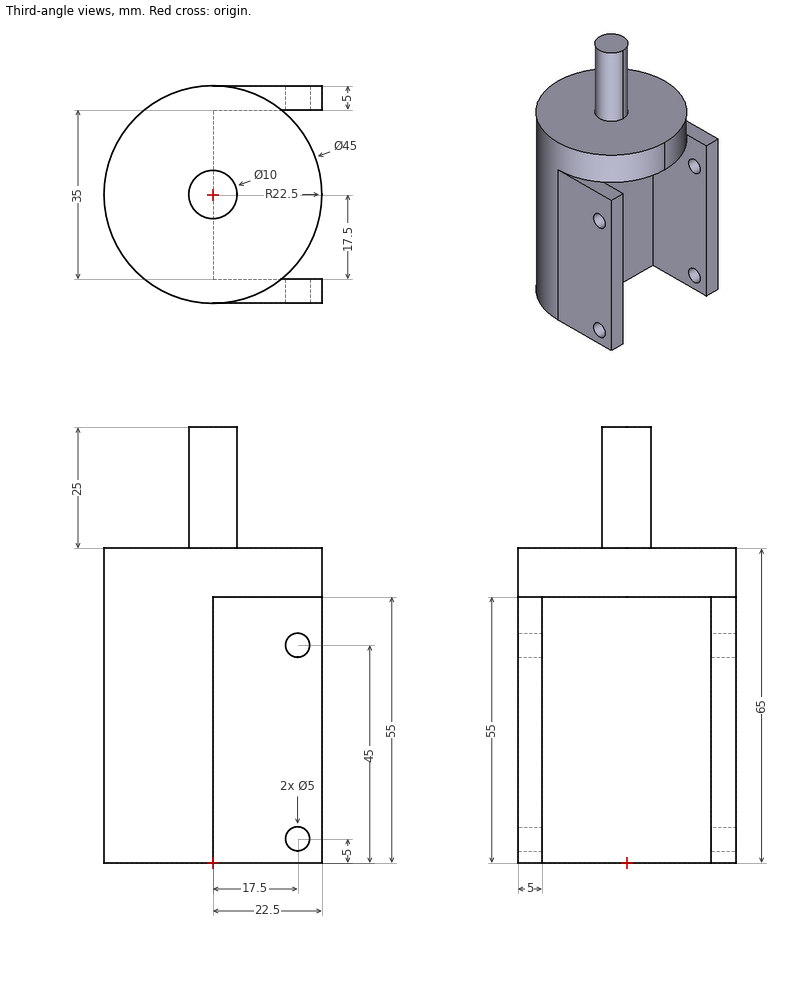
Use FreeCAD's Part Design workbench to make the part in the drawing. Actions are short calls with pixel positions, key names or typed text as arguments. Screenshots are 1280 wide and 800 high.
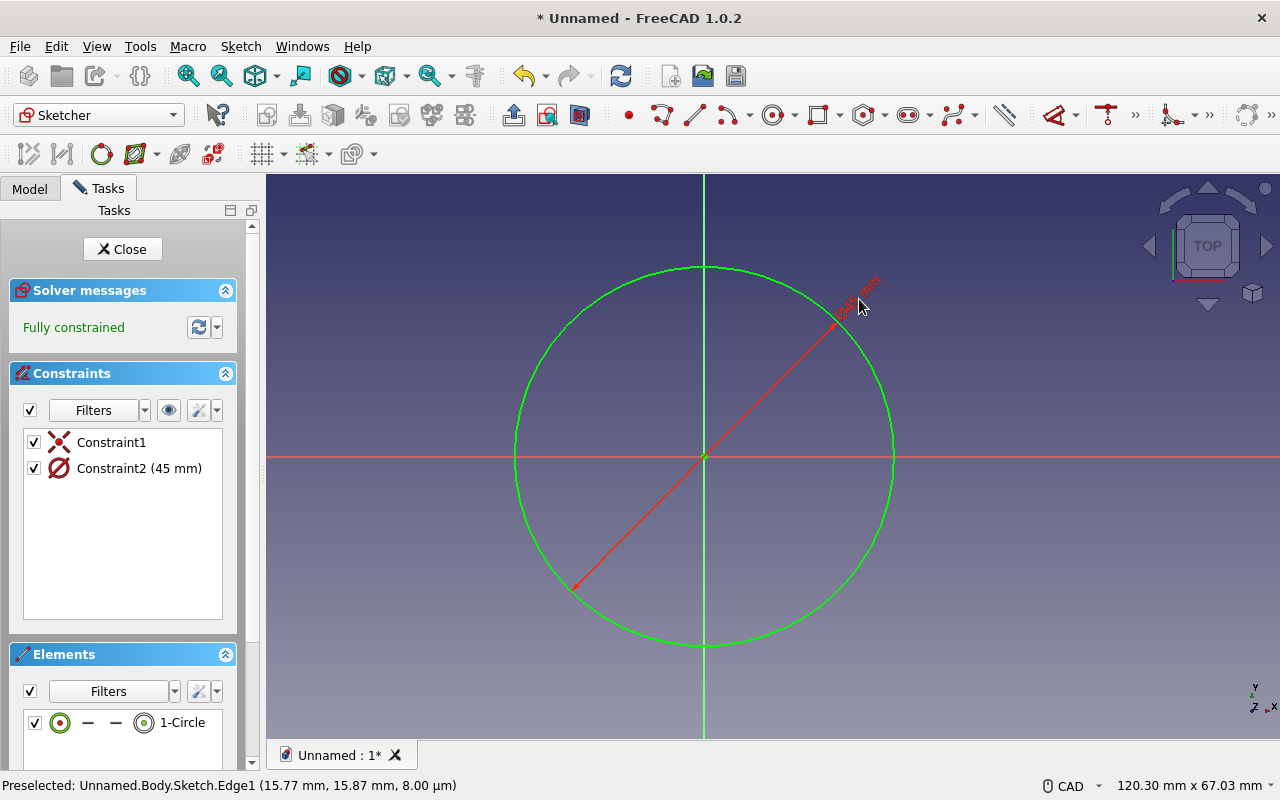
click(123, 249)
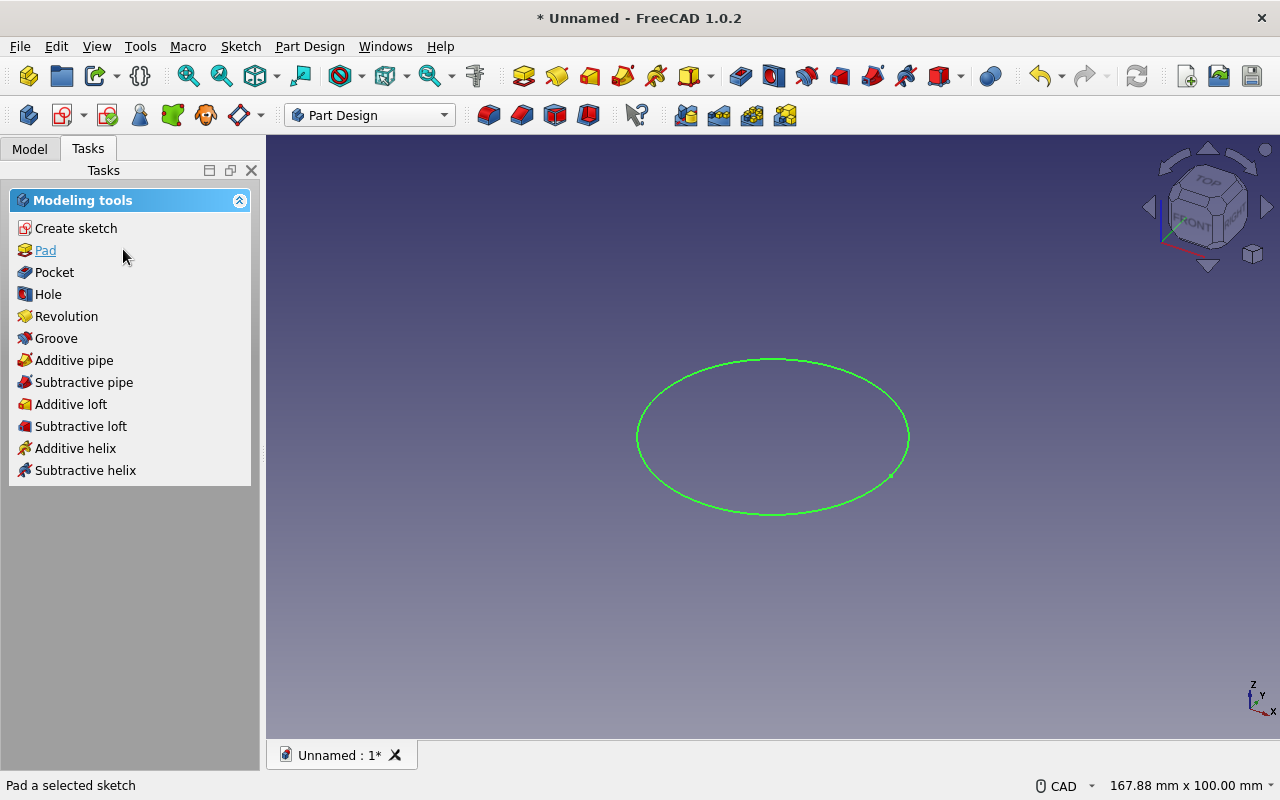
click(524, 76)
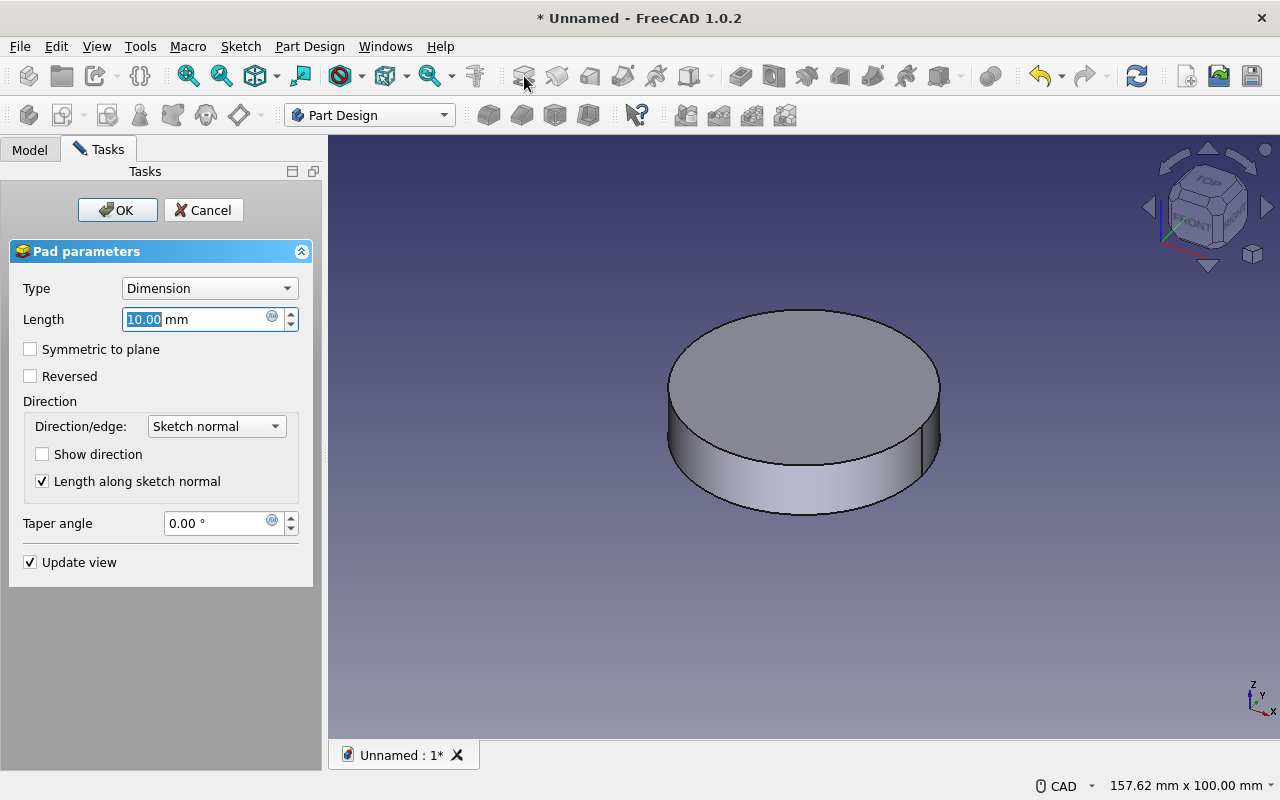
text(65)
key(Tab)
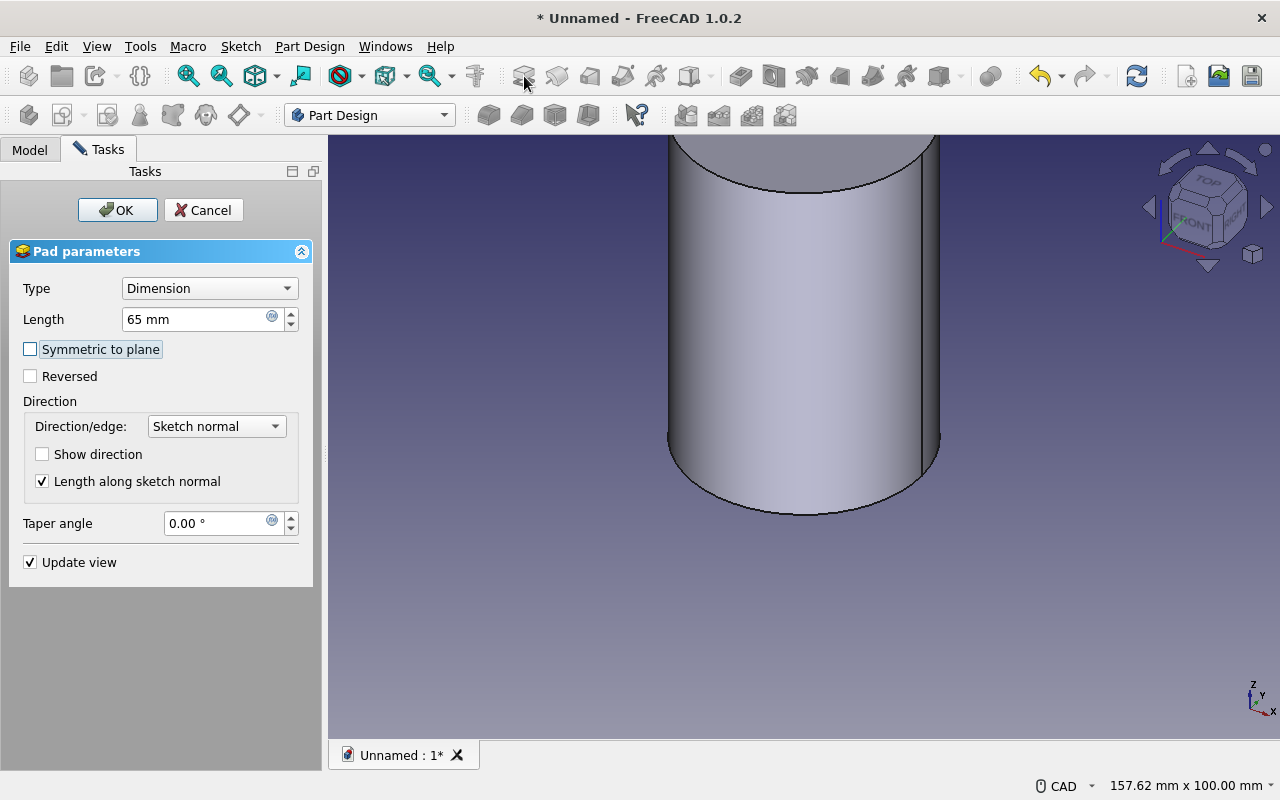
click(118, 210)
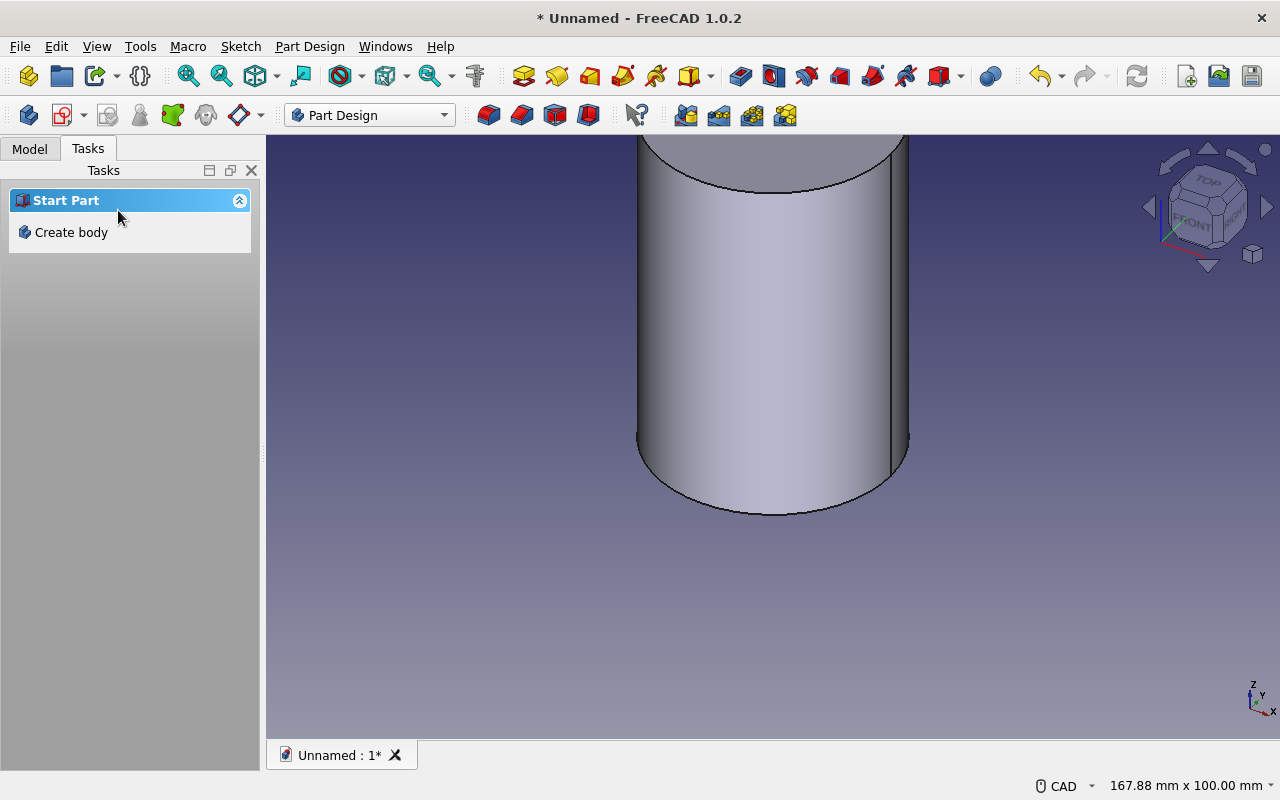
click(189, 76)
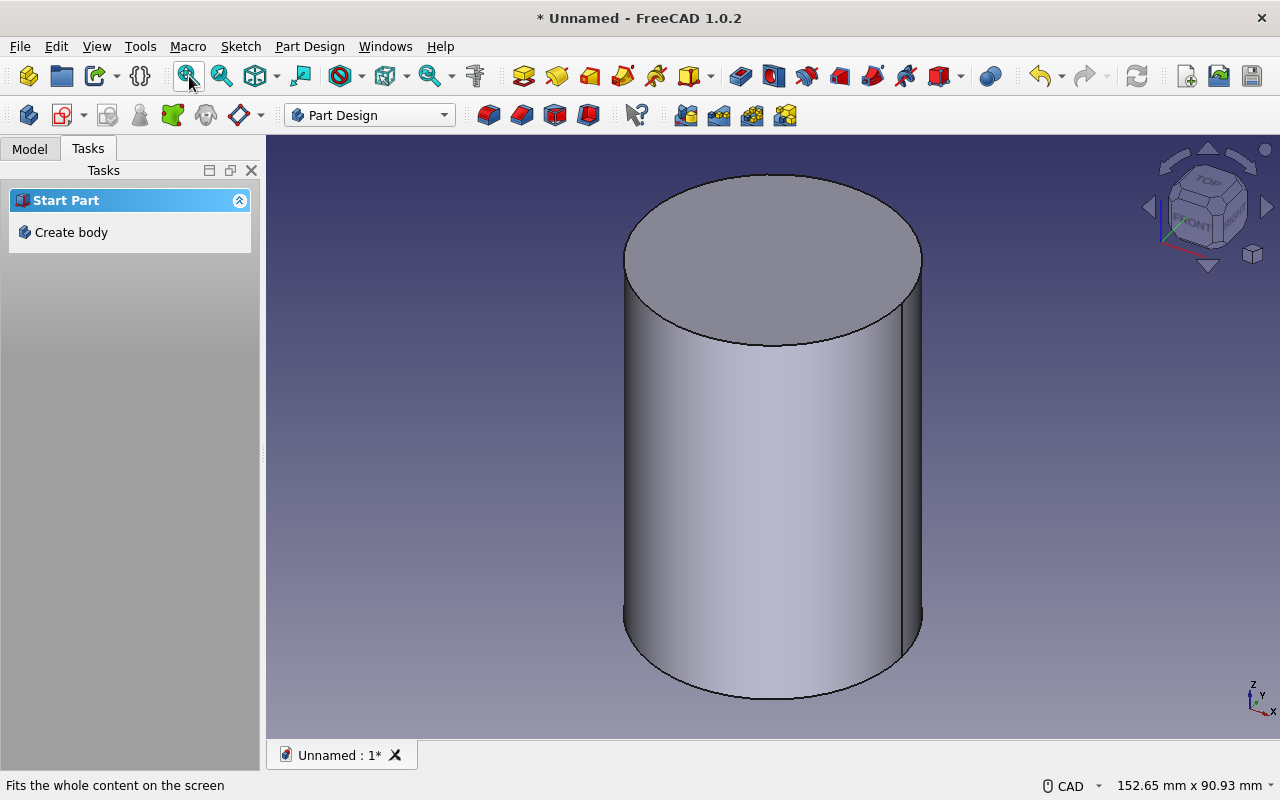
click(773, 259)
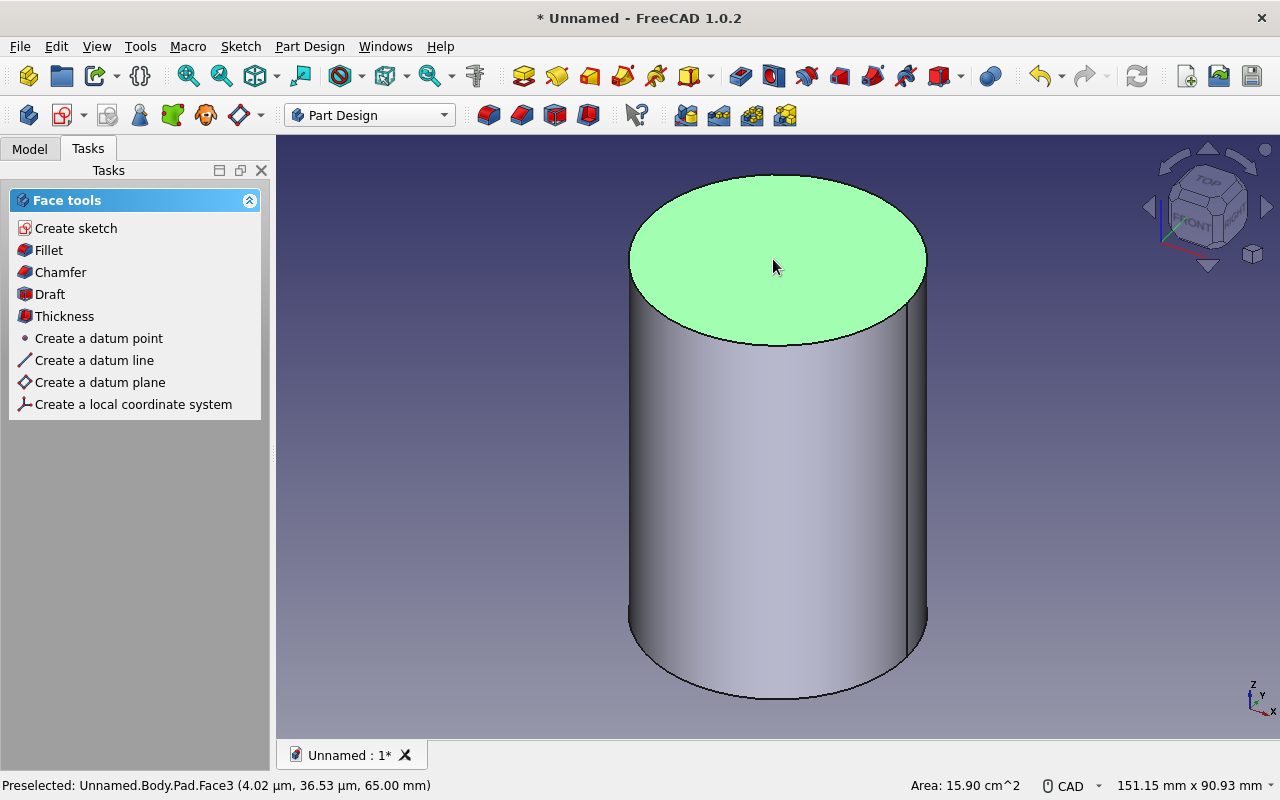
click(62, 116)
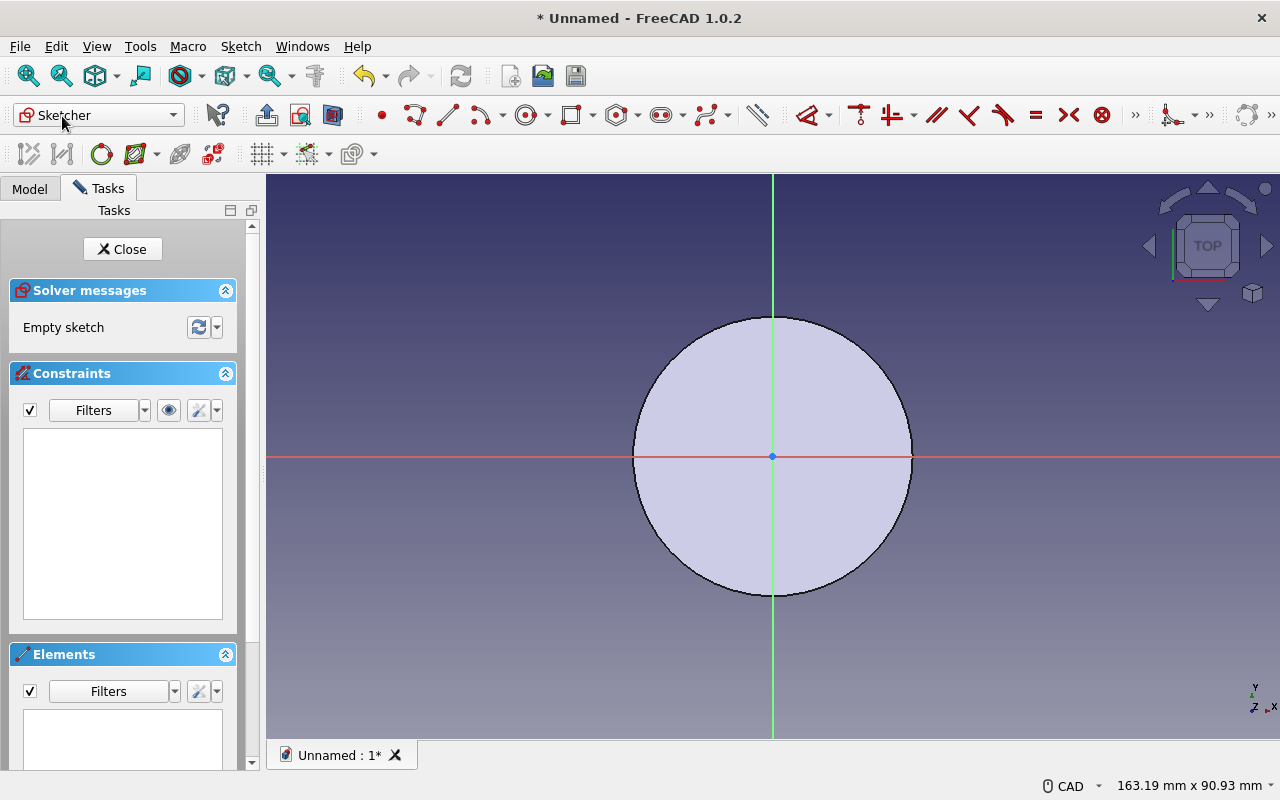
scroll(786, 456, up, 9)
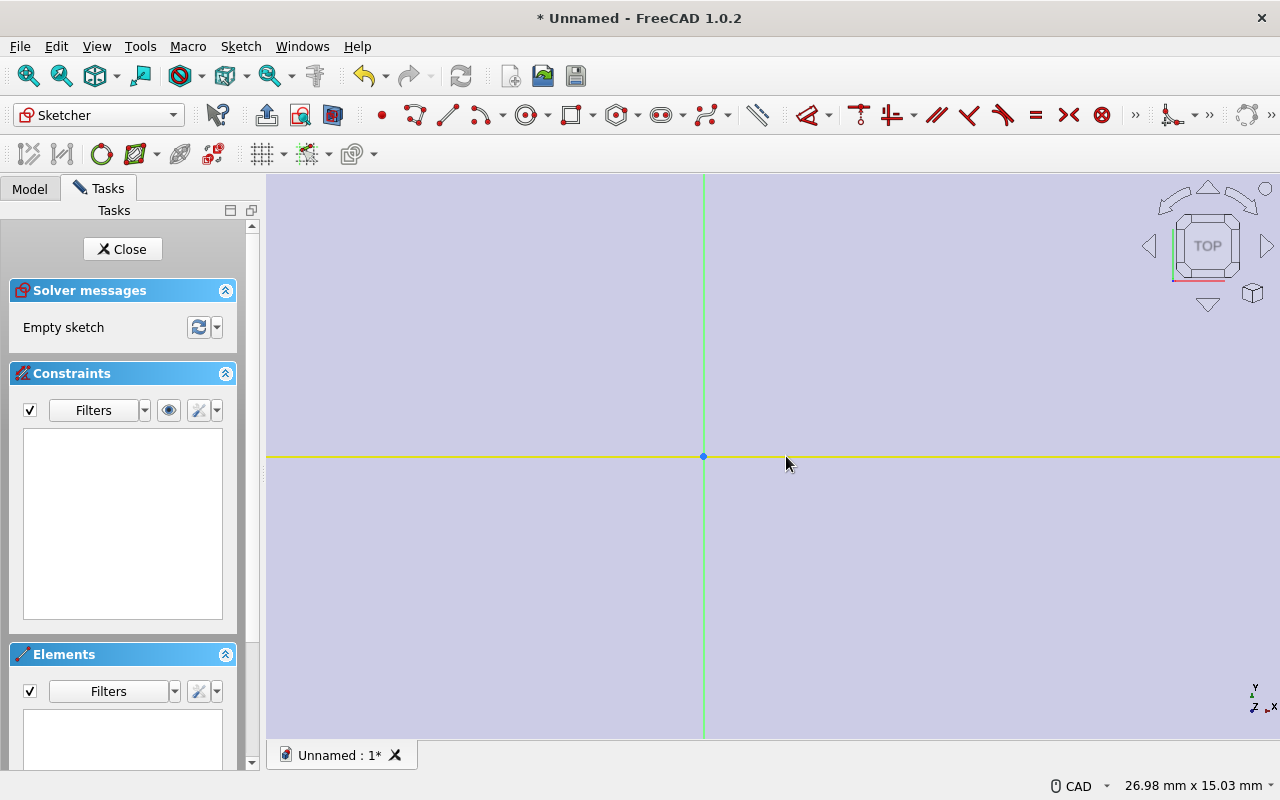
click(526, 116)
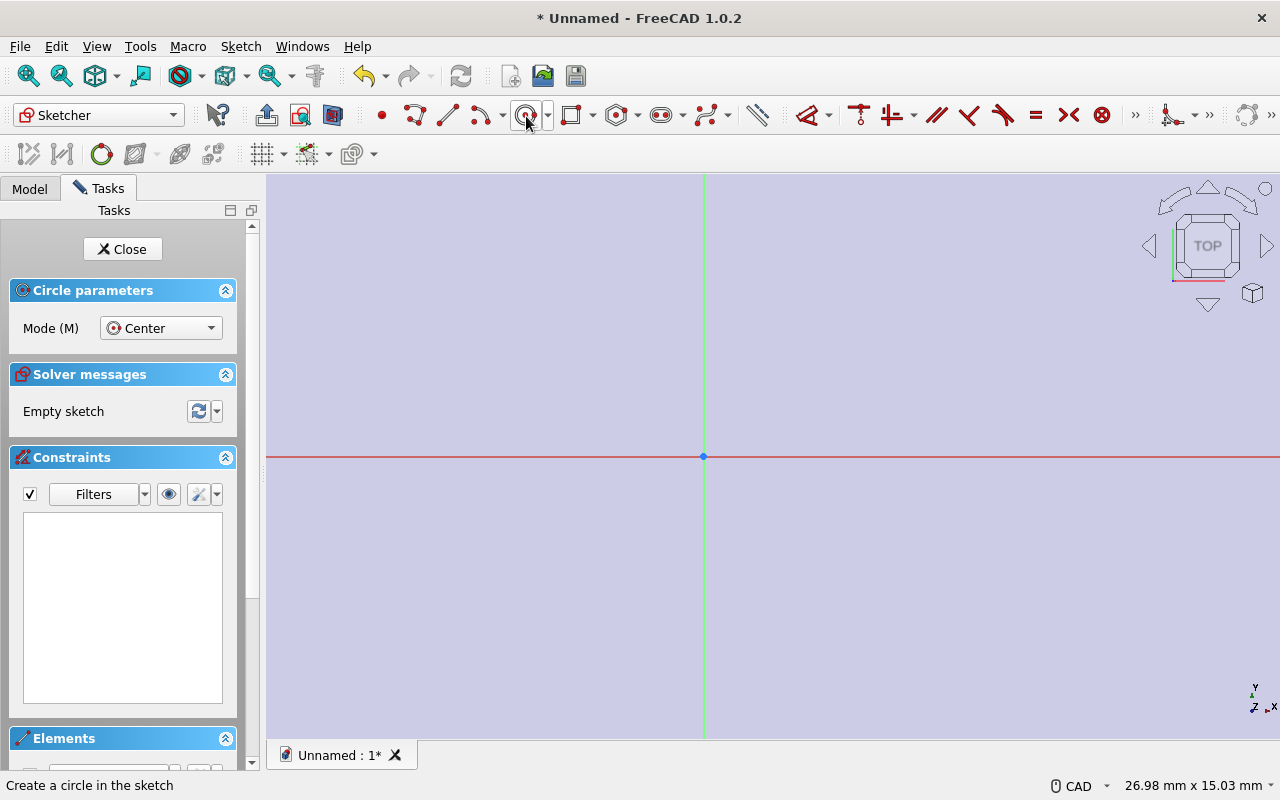
click(704, 456)
click(837, 324)
key(Escape)